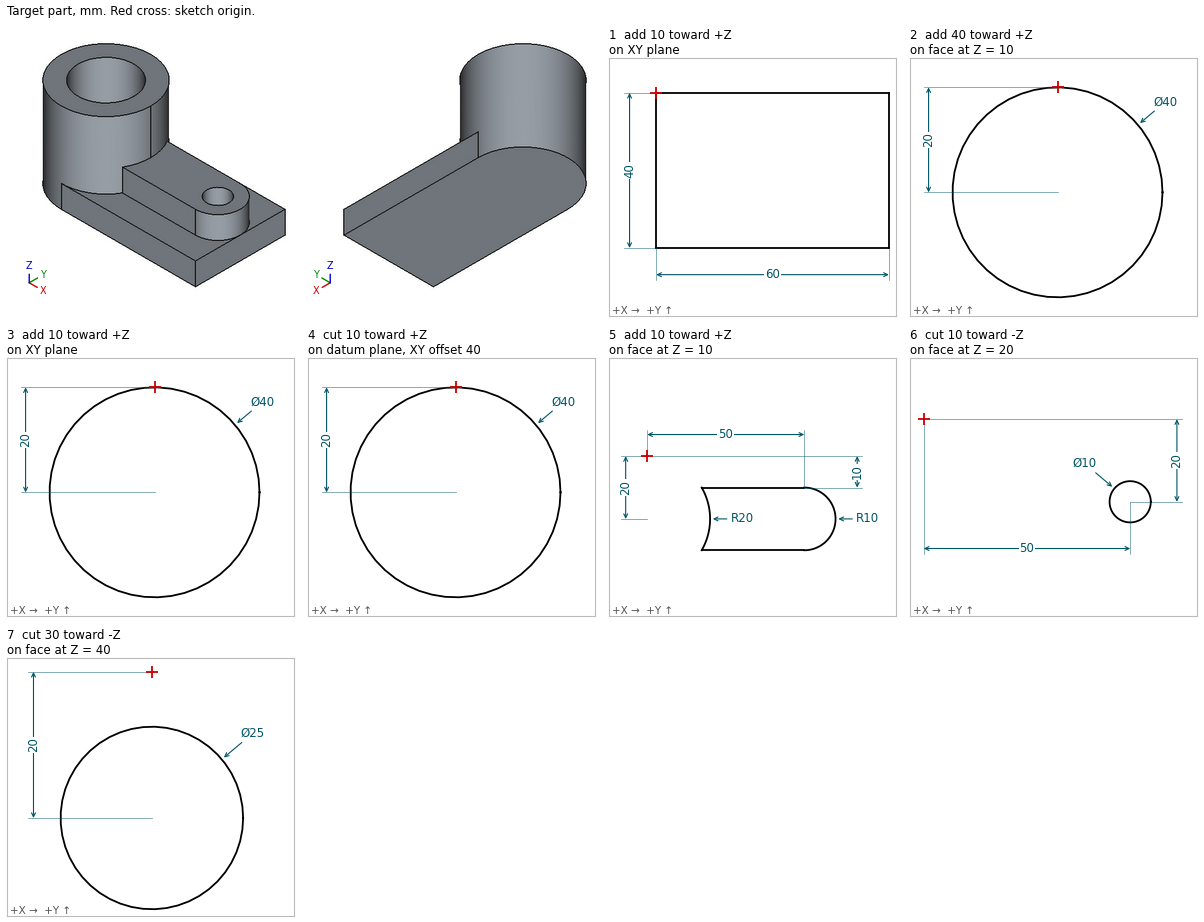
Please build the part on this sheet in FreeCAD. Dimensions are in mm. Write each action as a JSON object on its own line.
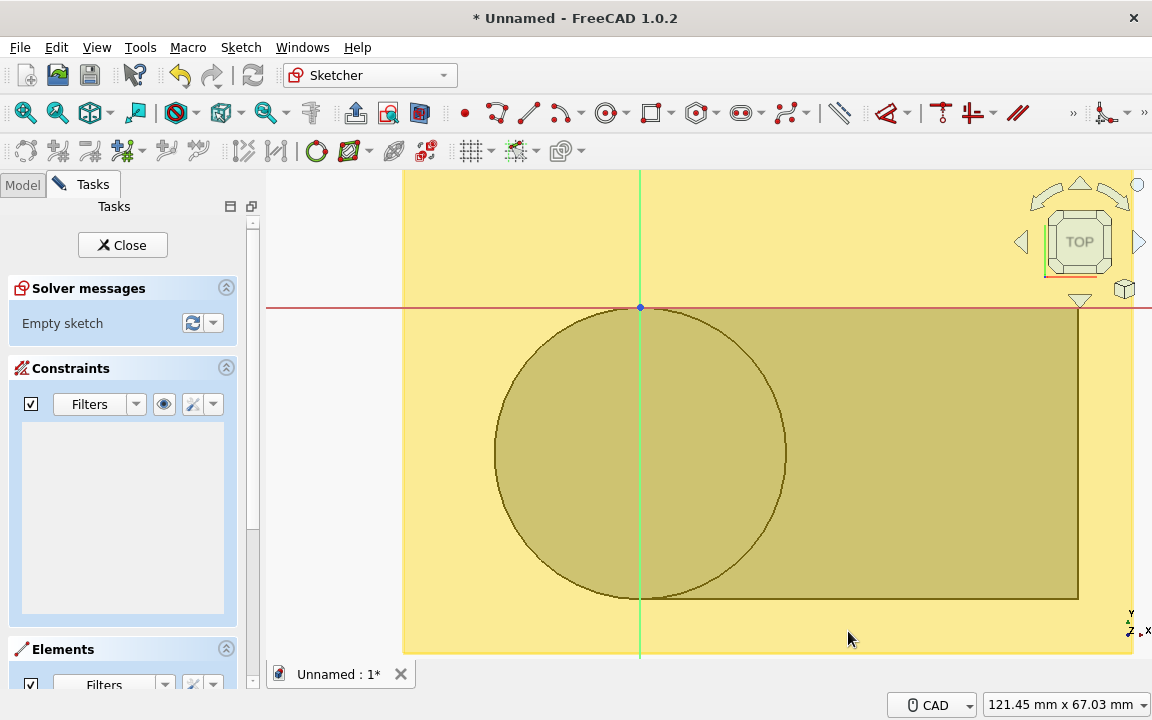
{"action": "left_click", "coordinate": [606, 114]}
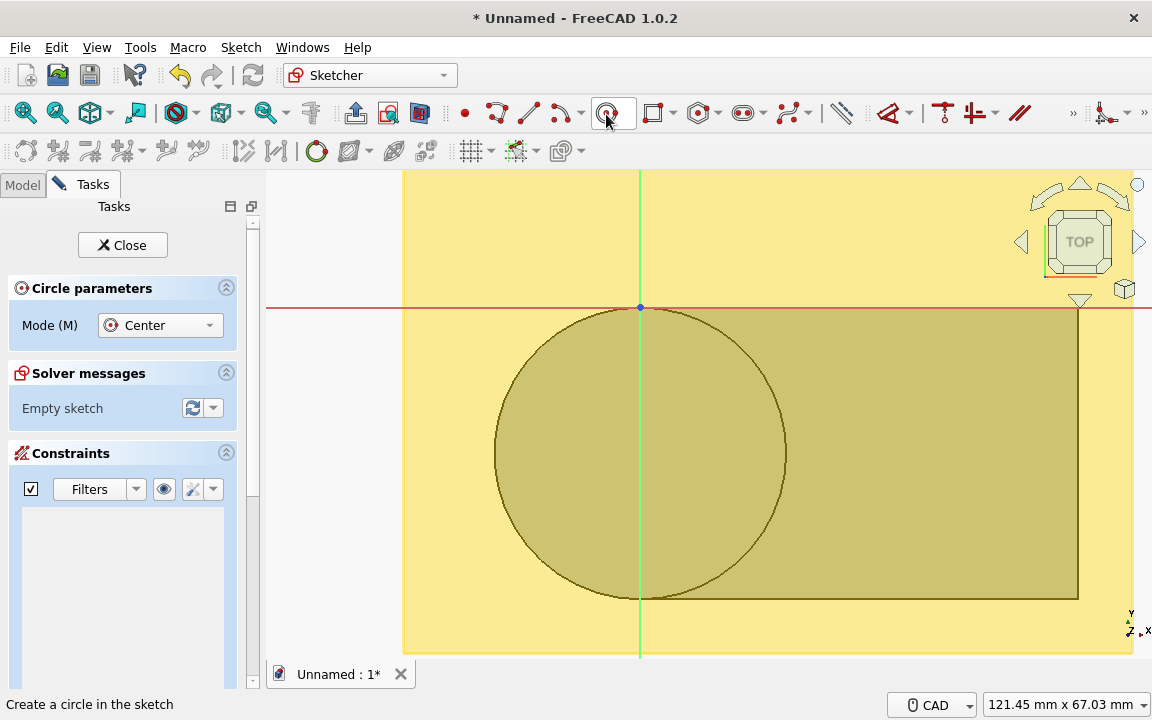
{"action": "left_click", "coordinate": [640, 453]}
{"action": "left_click", "coordinate": [743, 350]}
{"action": "key", "text": "Escape"}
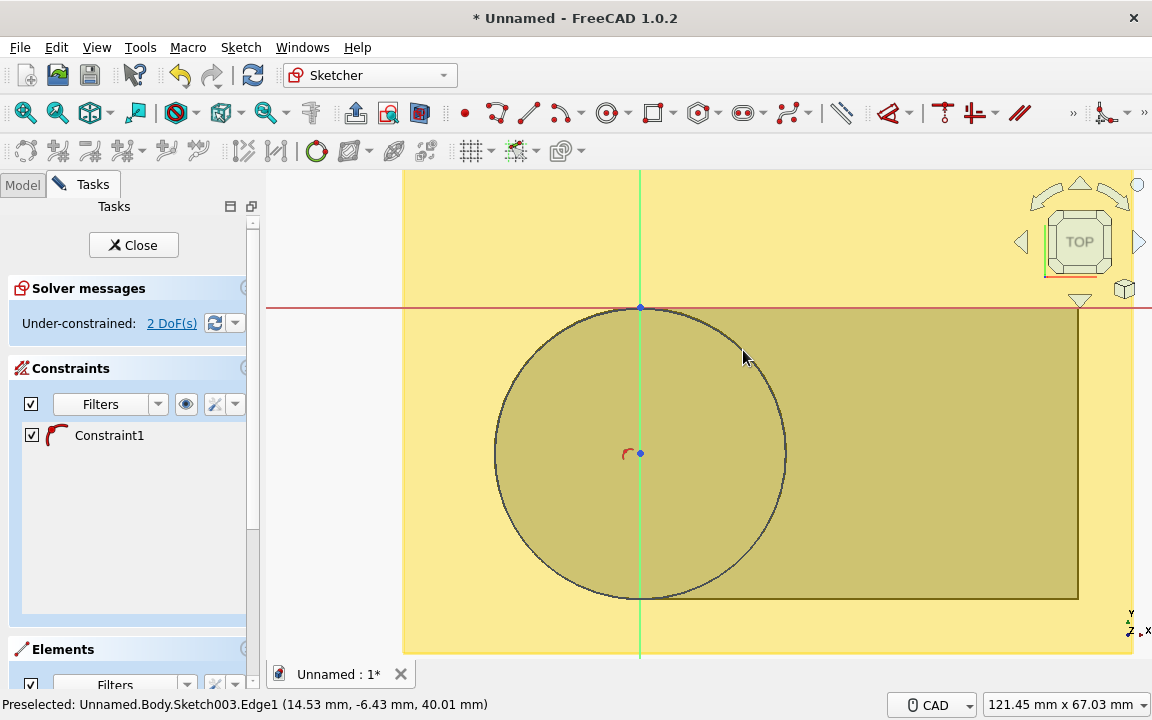
{"action": "left_click", "coordinate": [888, 114]}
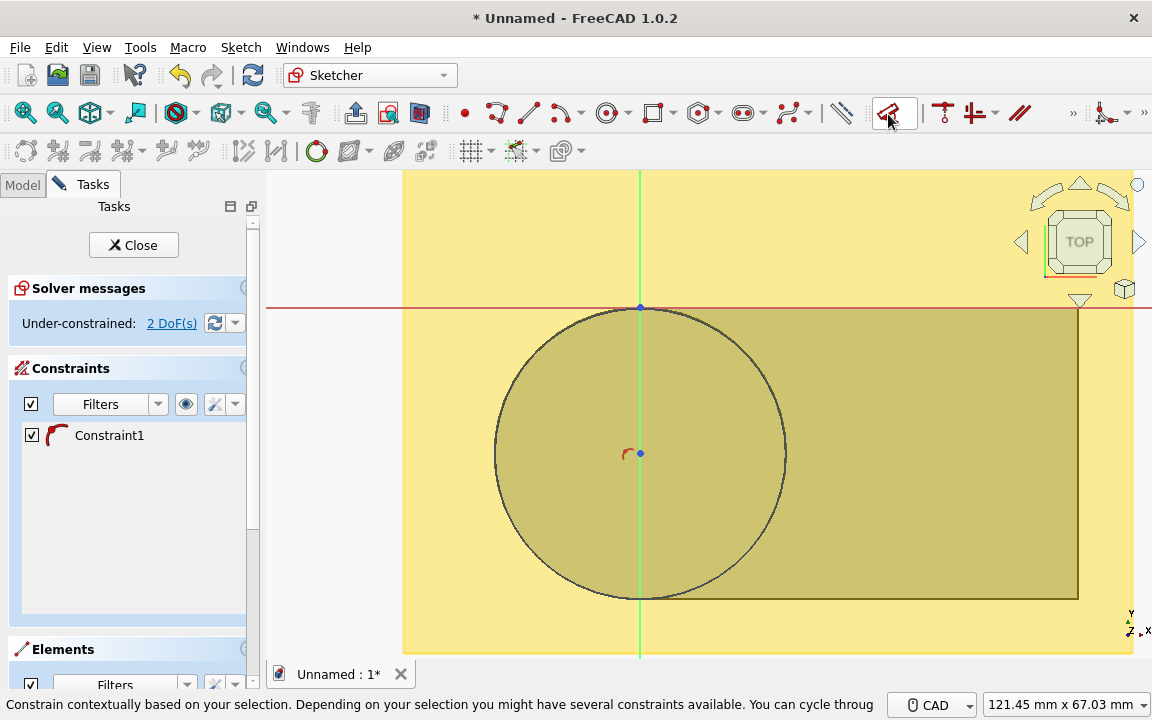
{"action": "left_click", "coordinate": [743, 351]}
{"action": "left_click", "coordinate": [766, 328]}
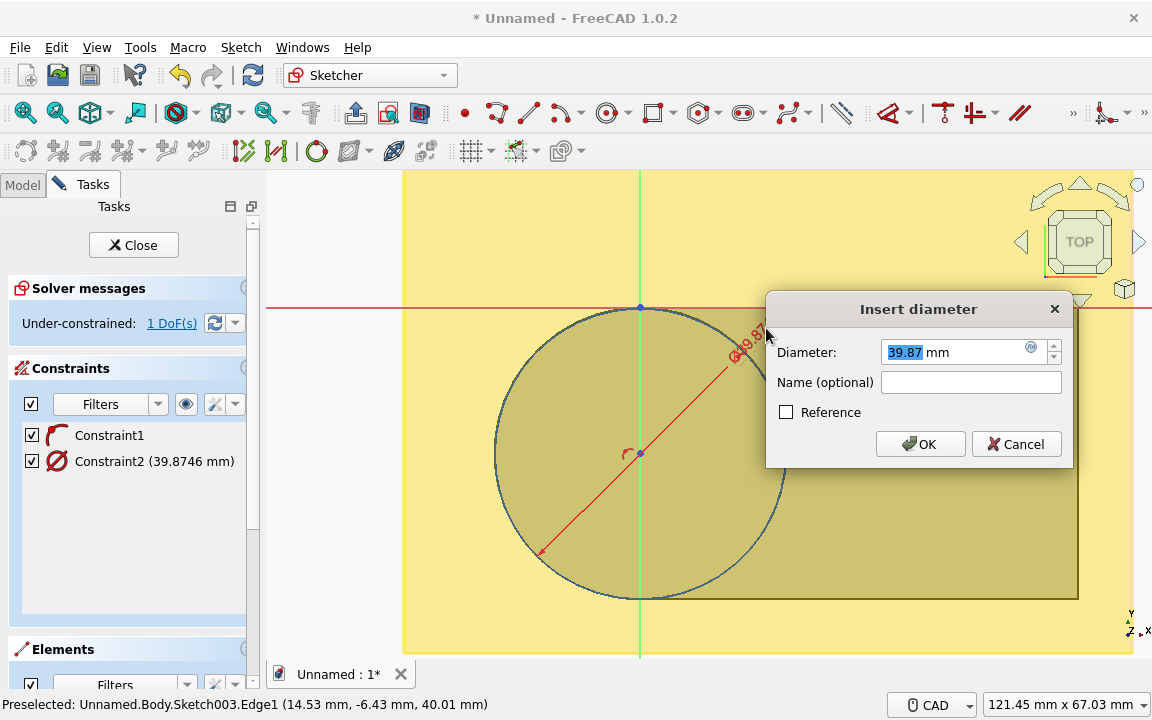
{"action": "type", "text": "40"}
{"action": "key", "text": "Return"}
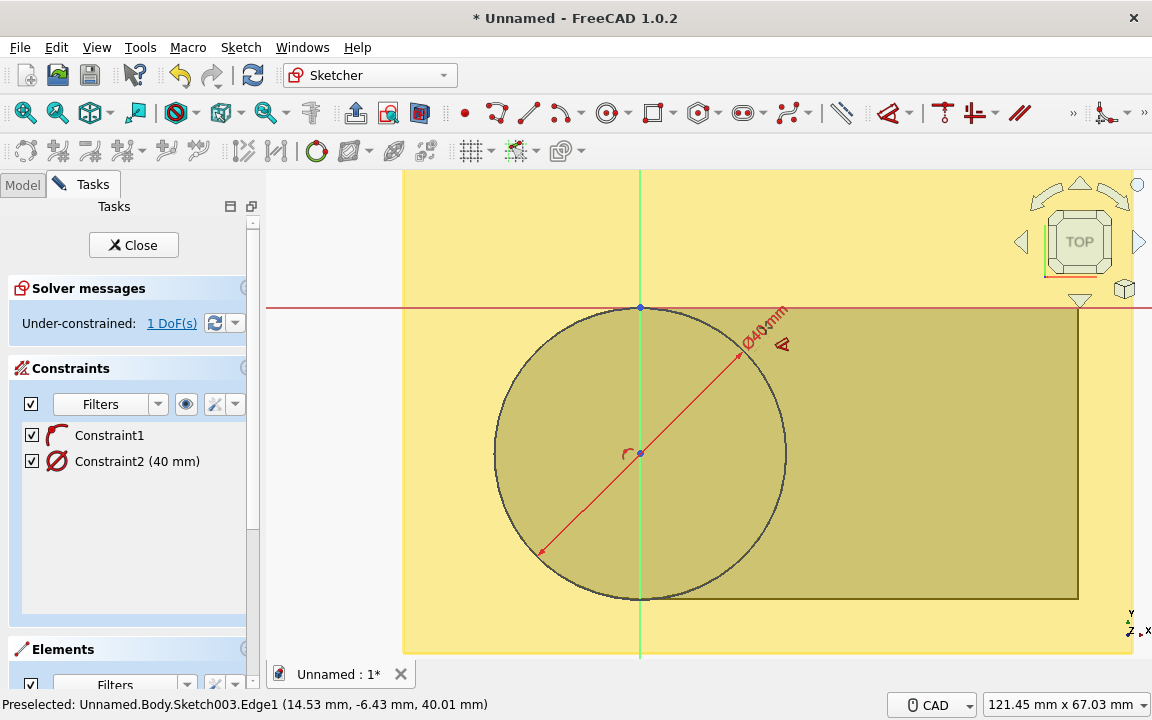
{"action": "left_click", "coordinate": [640, 454]}
{"action": "left_click", "coordinate": [674, 381]}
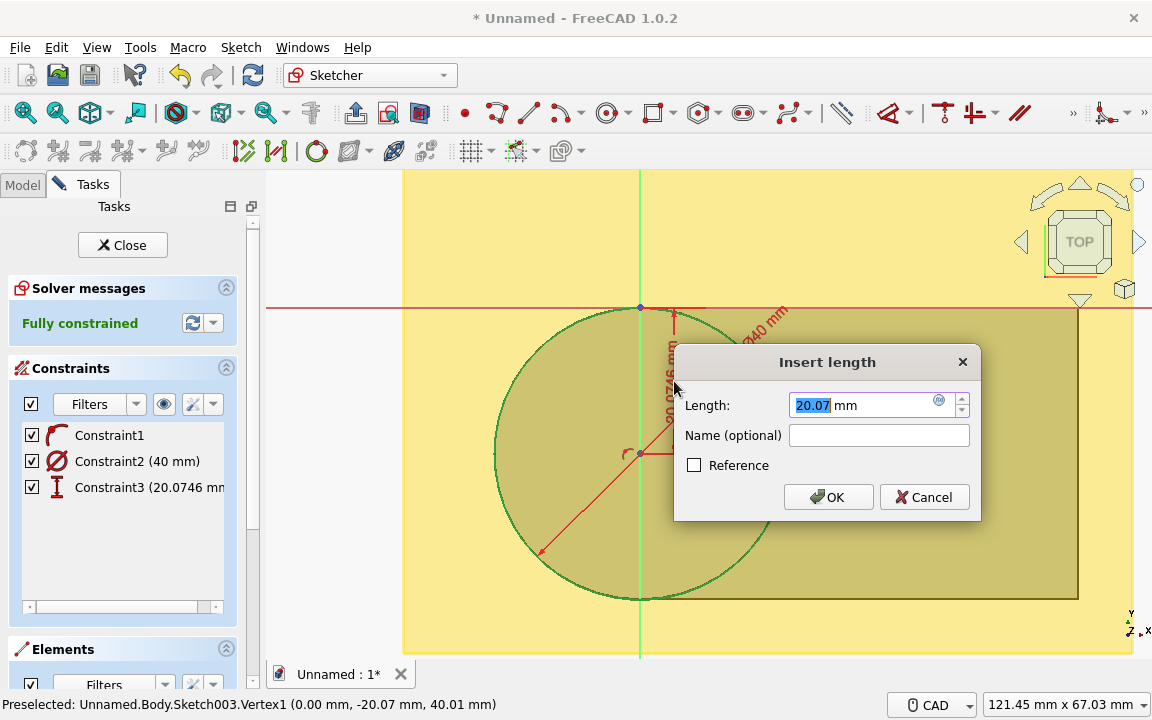
{"action": "type", "text": "20"}
{"action": "key", "text": "Return"}
{"action": "key", "text": "Escape"}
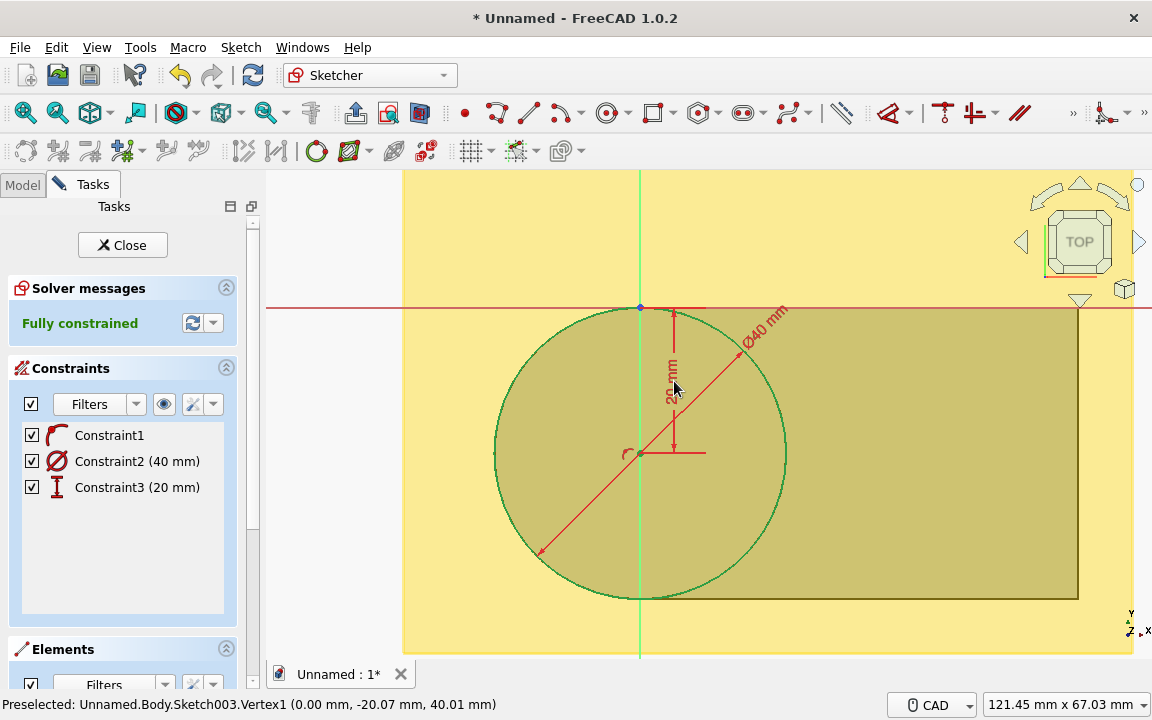
{"action": "left_click", "coordinate": [123, 245]}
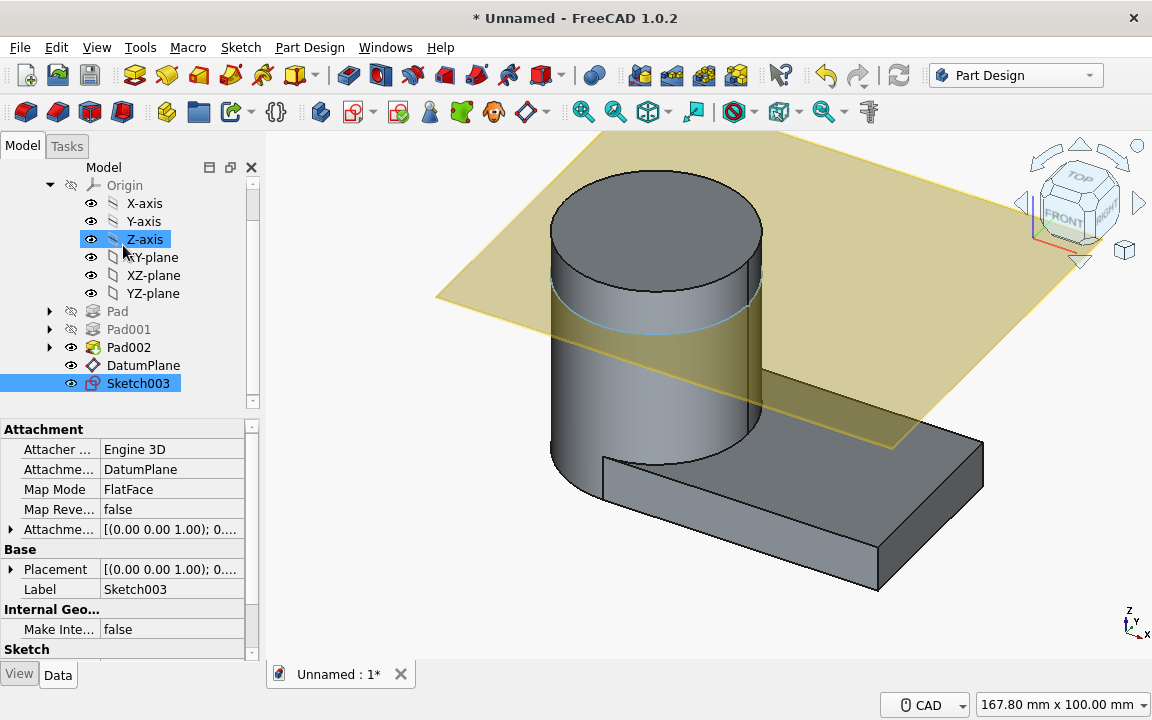
{"action": "left_click", "coordinate": [350, 76]}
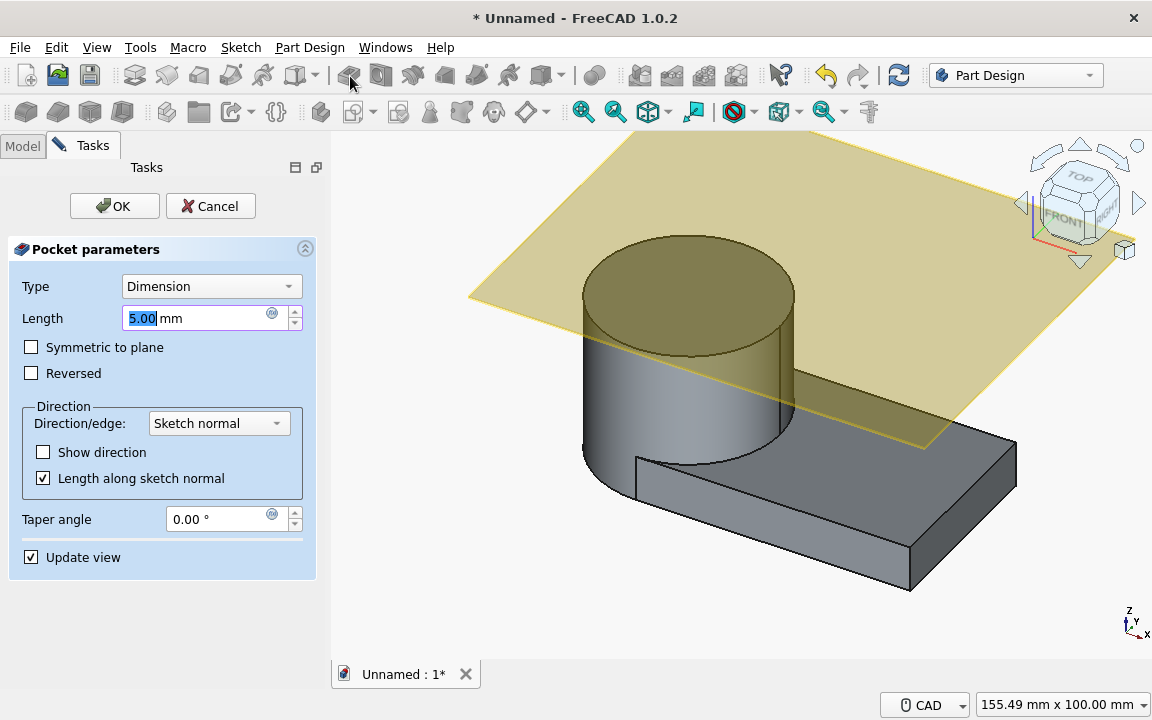
{"action": "type", "text": "10"}
{"action": "key", "text": "Tab"}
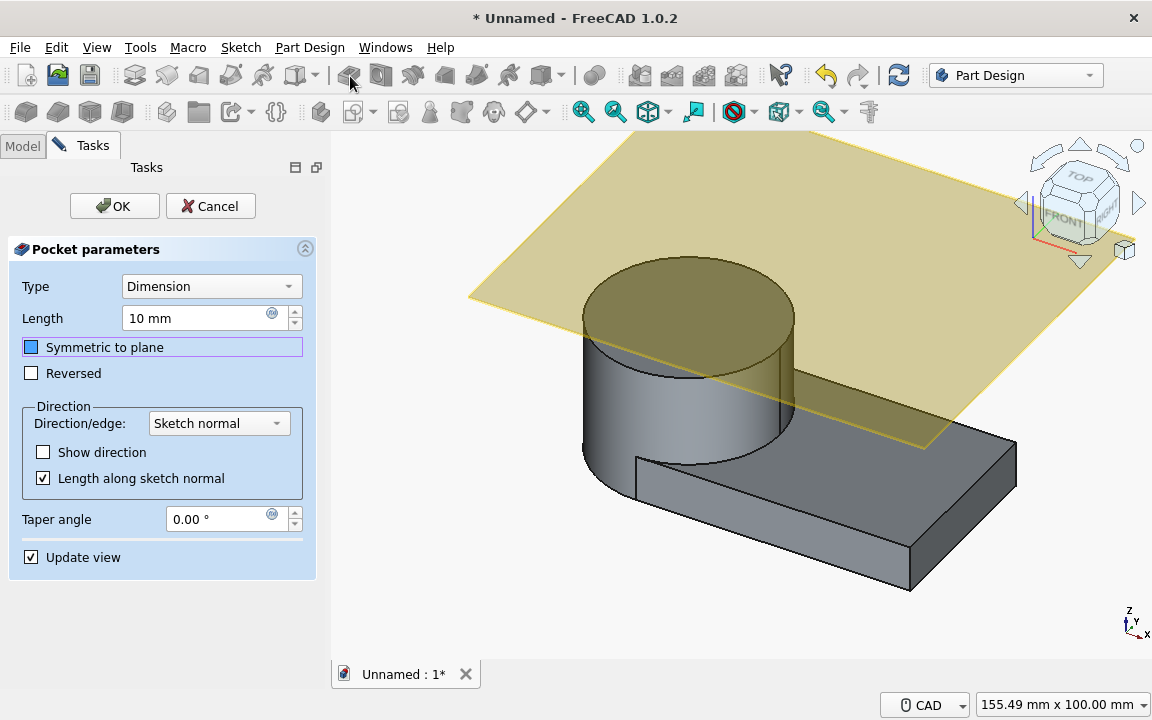
{"action": "left_click", "coordinate": [30, 373]}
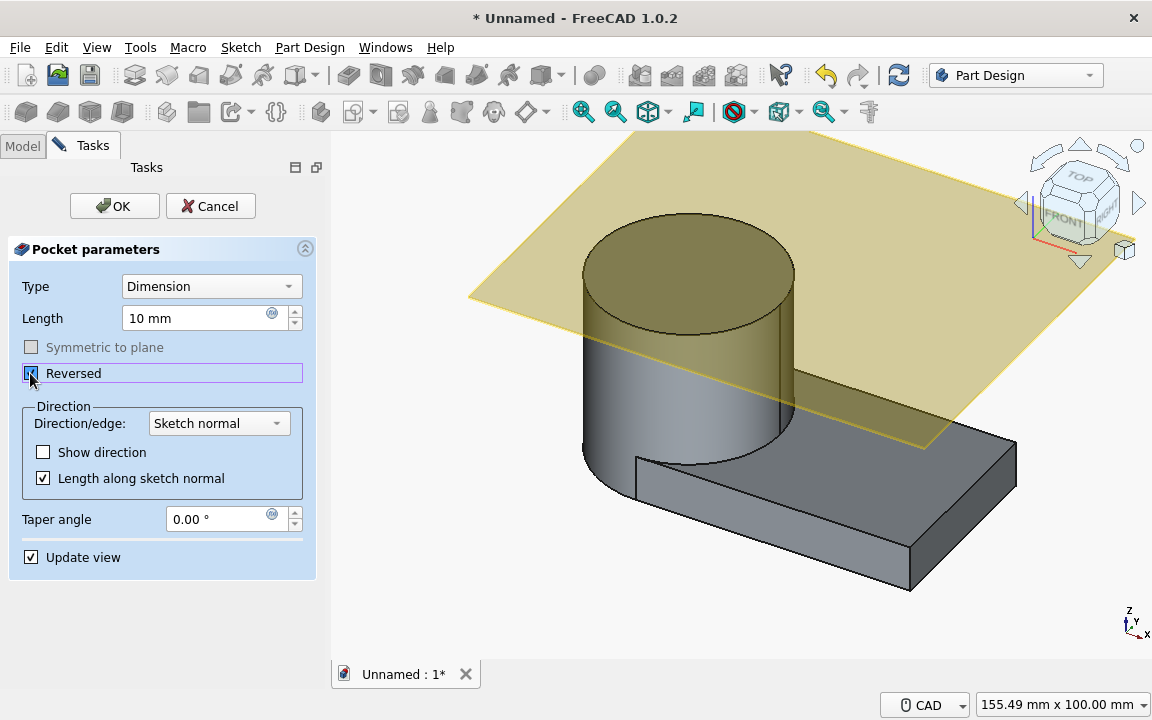
{"action": "left_click", "coordinate": [115, 206]}